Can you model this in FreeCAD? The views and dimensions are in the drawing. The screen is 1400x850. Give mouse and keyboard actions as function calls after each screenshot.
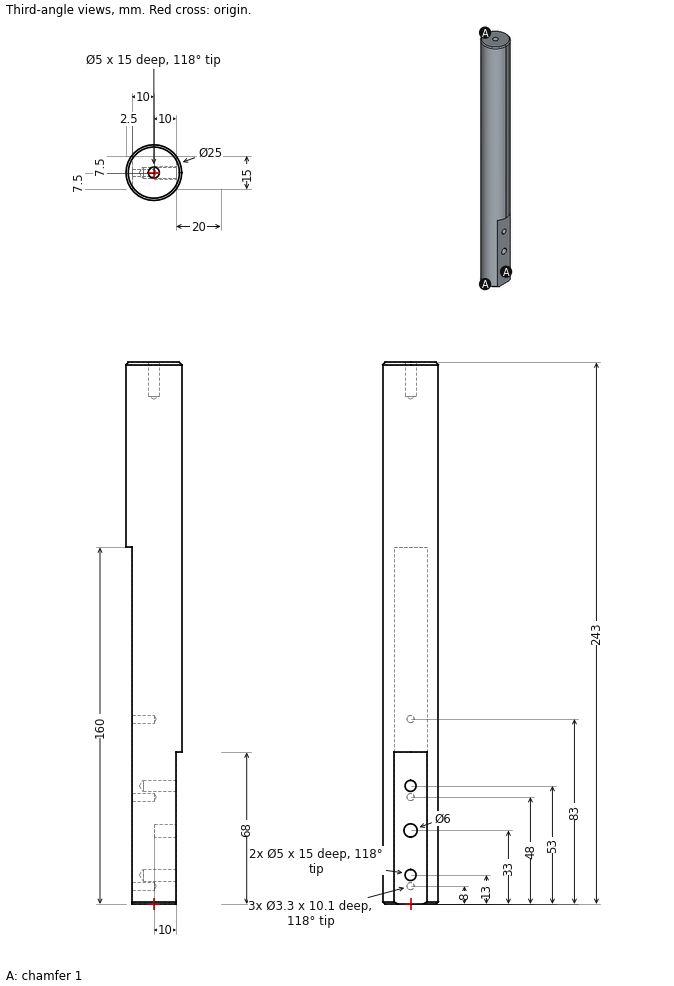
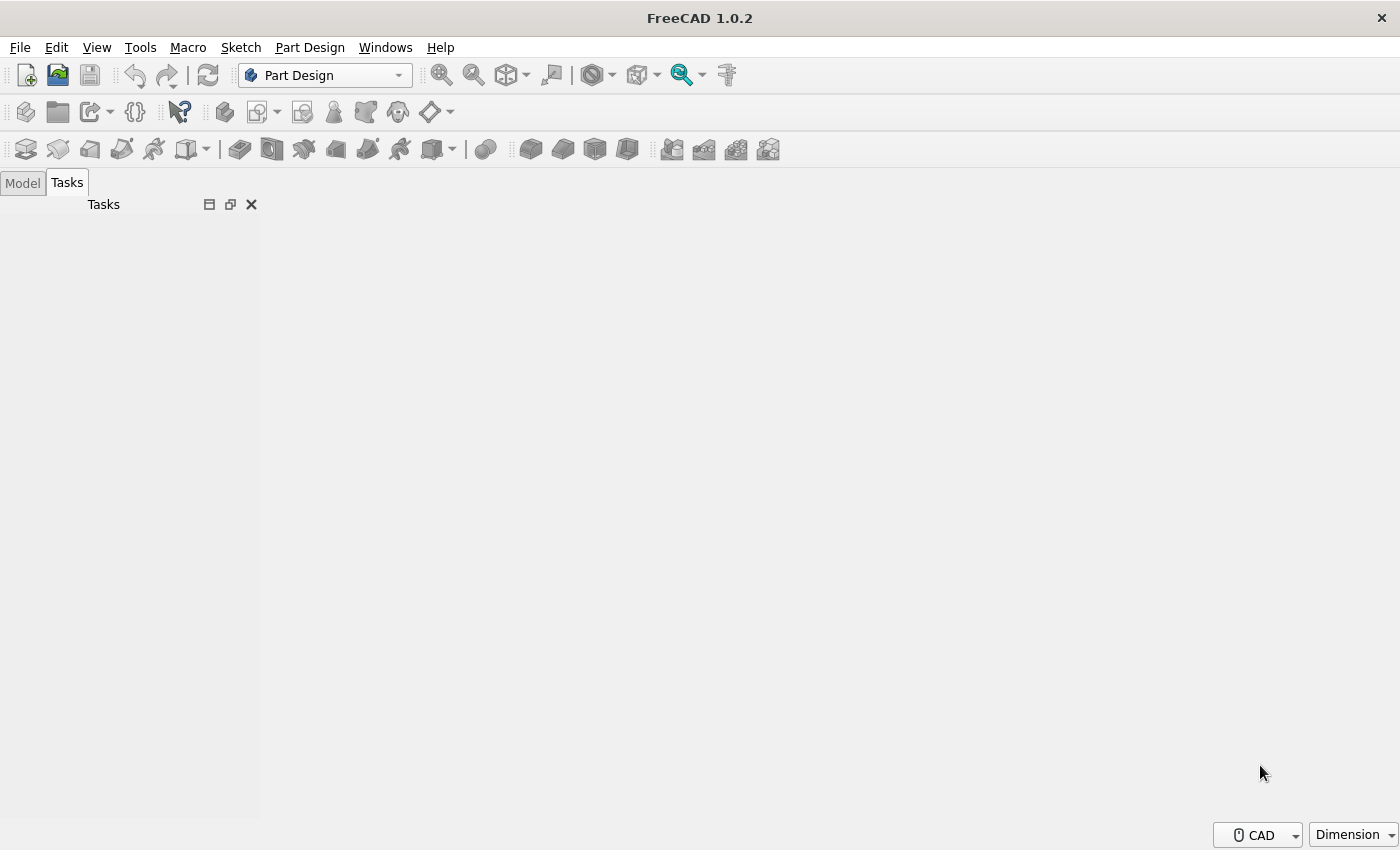
click(26, 76)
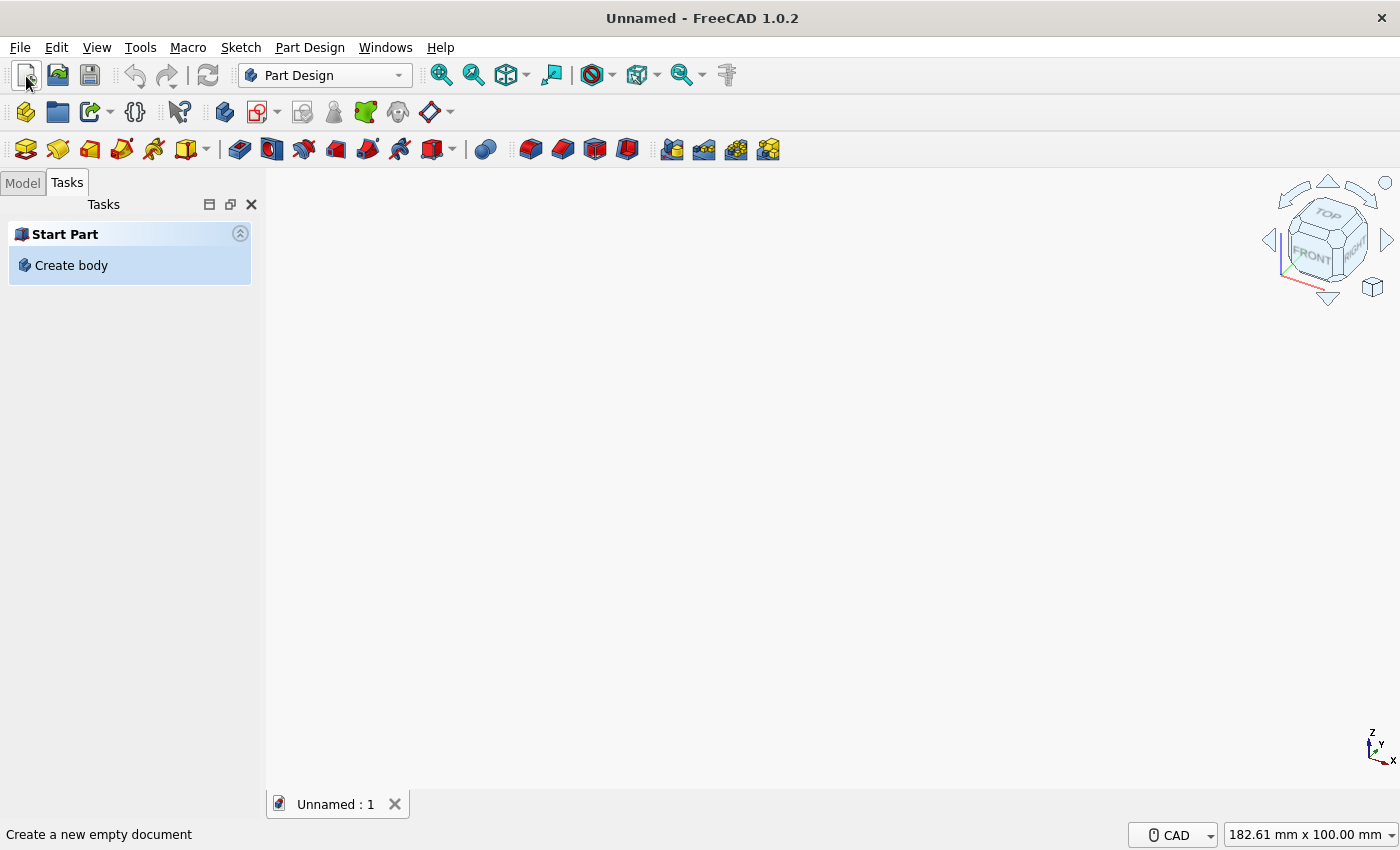
click(258, 112)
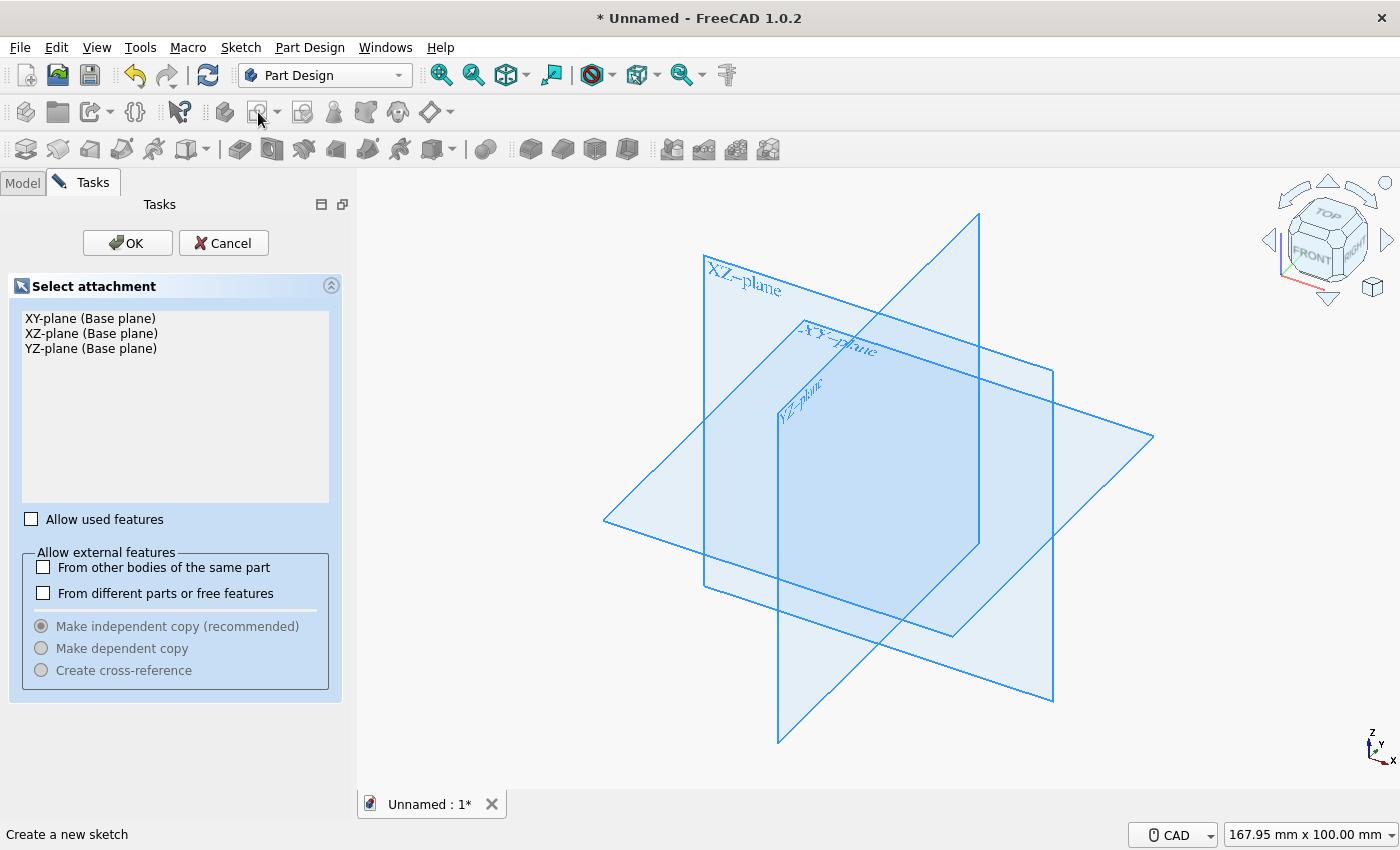
click(82, 318)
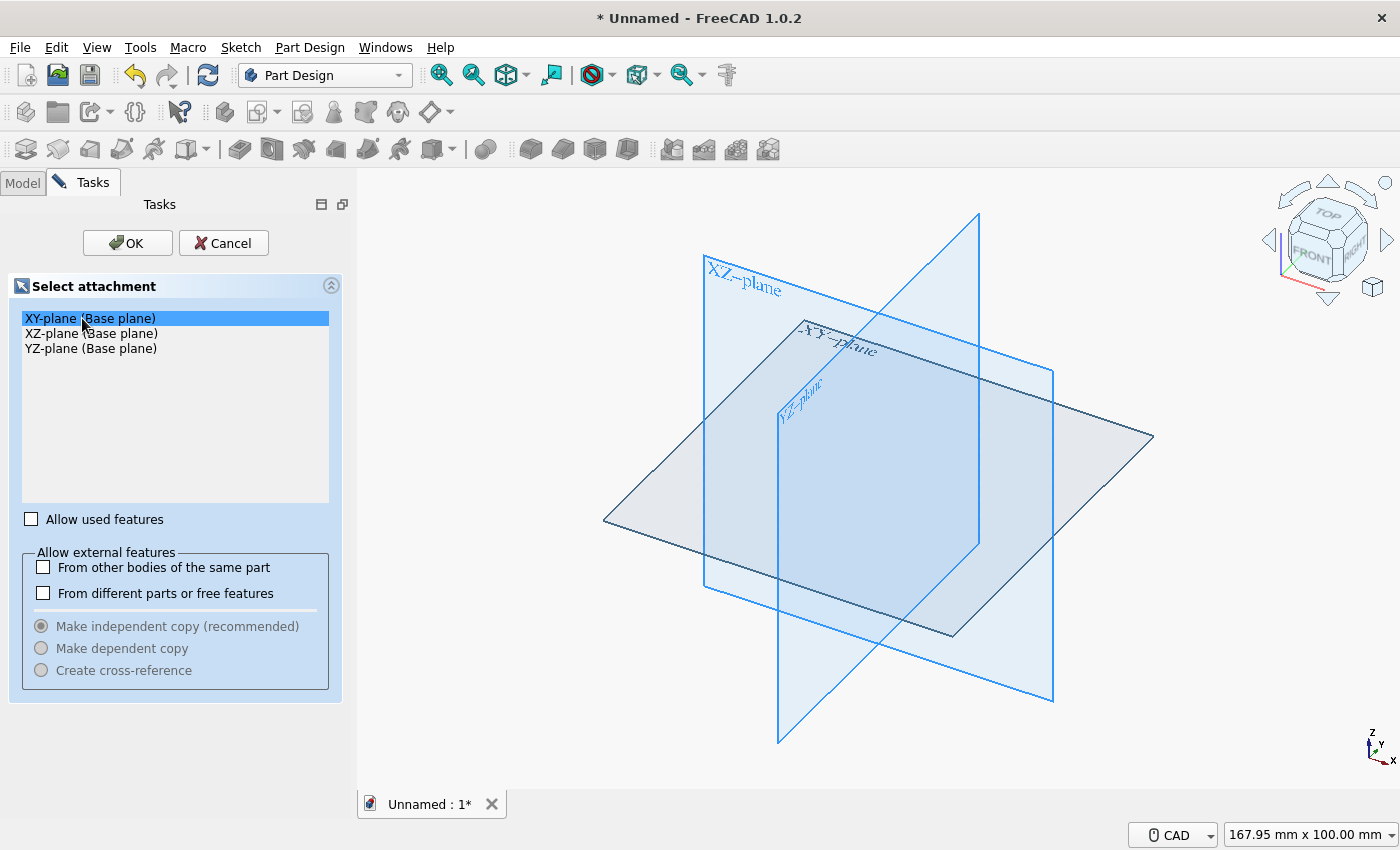
click(128, 243)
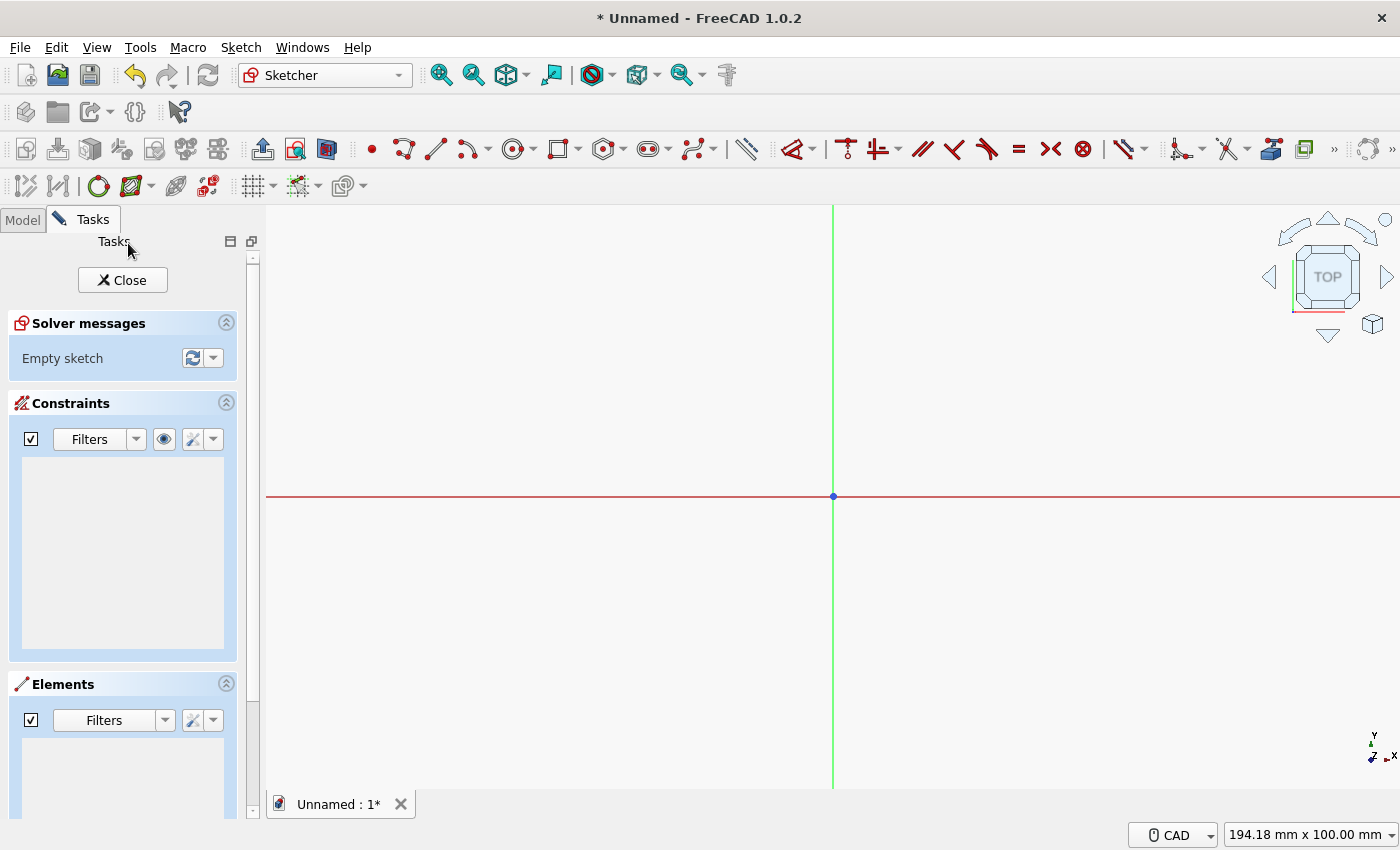
scroll(873, 497, up, 5)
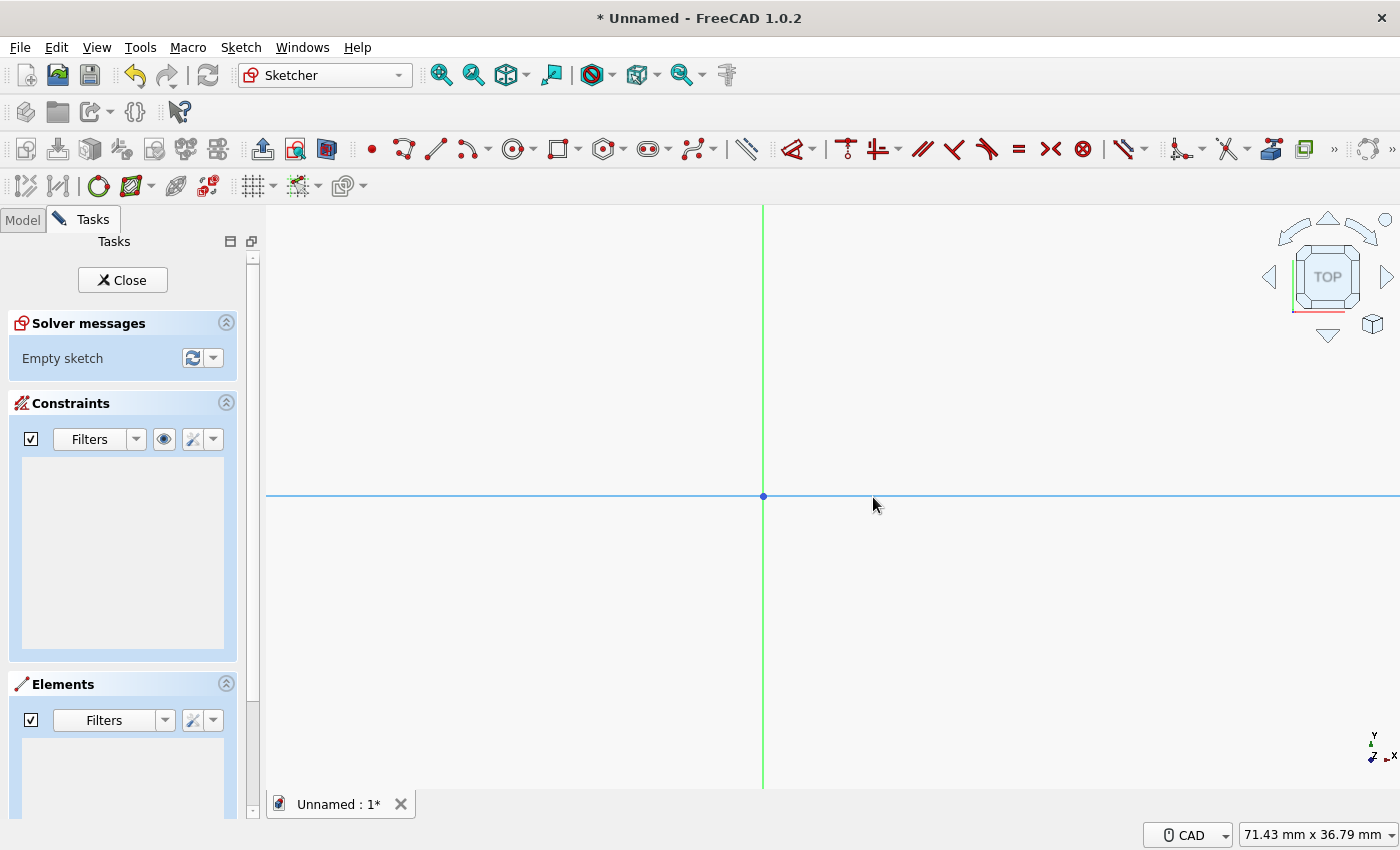
key(g)
key(c)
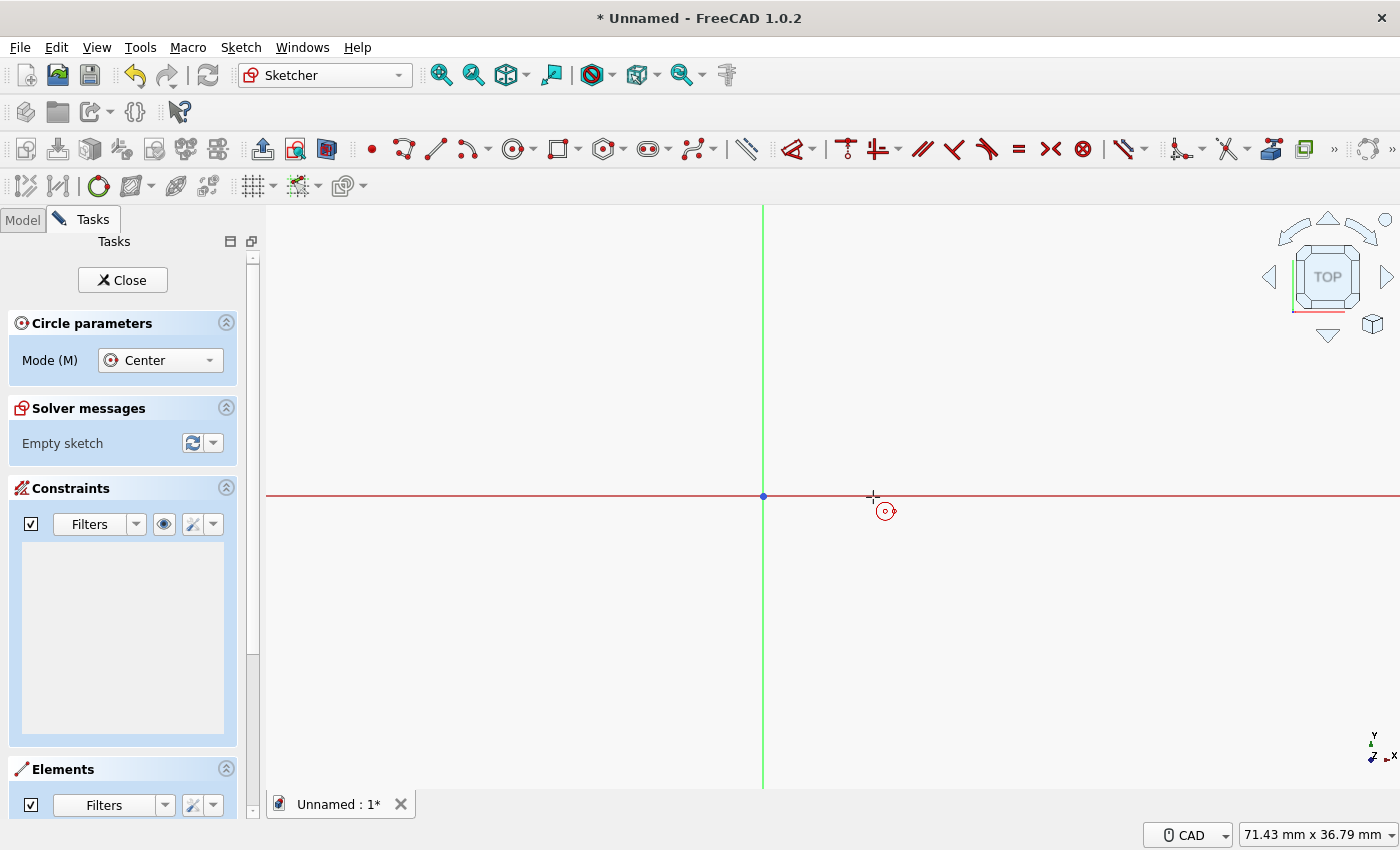
click(763, 496)
click(904, 356)
key(Escape)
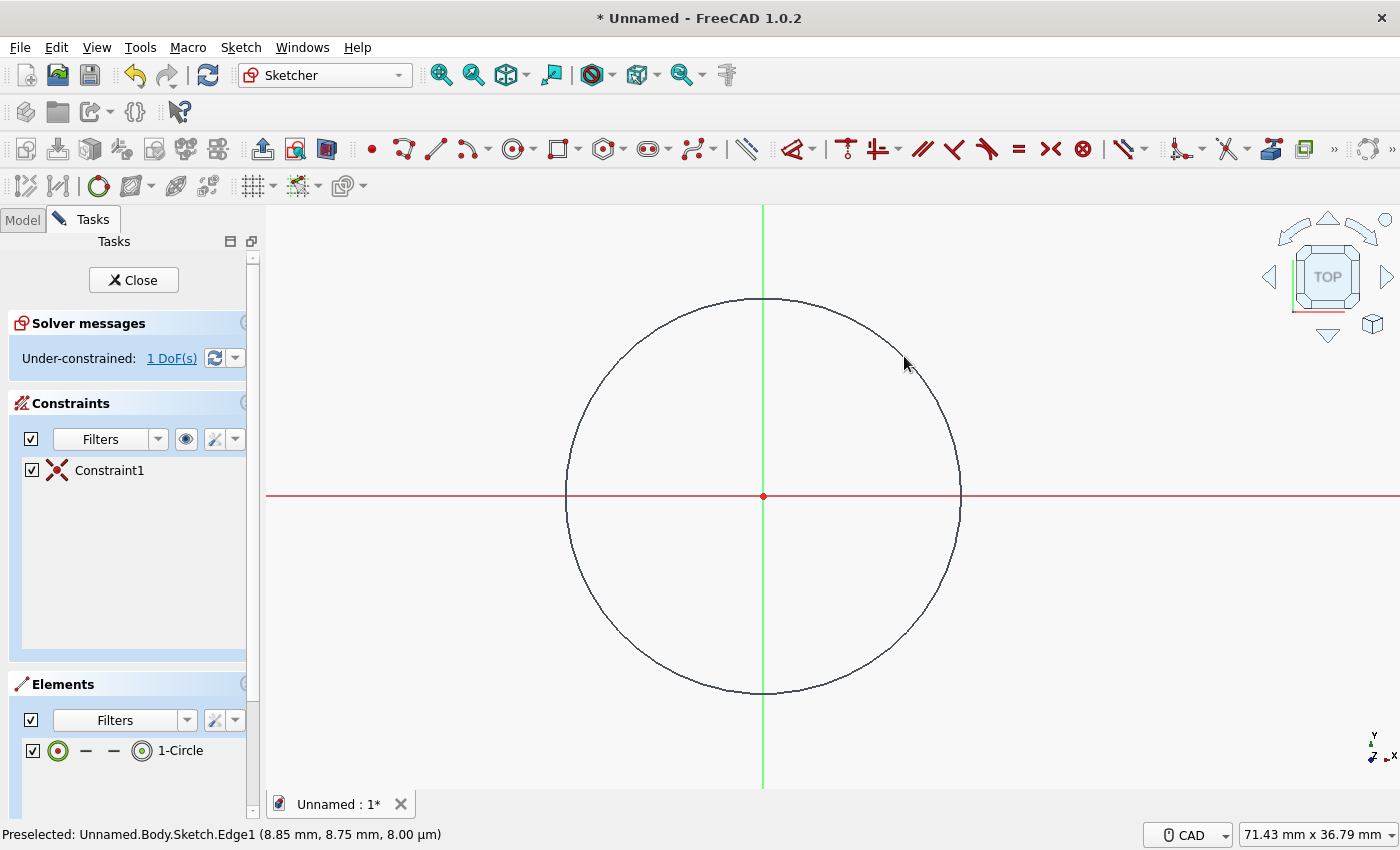
key(d)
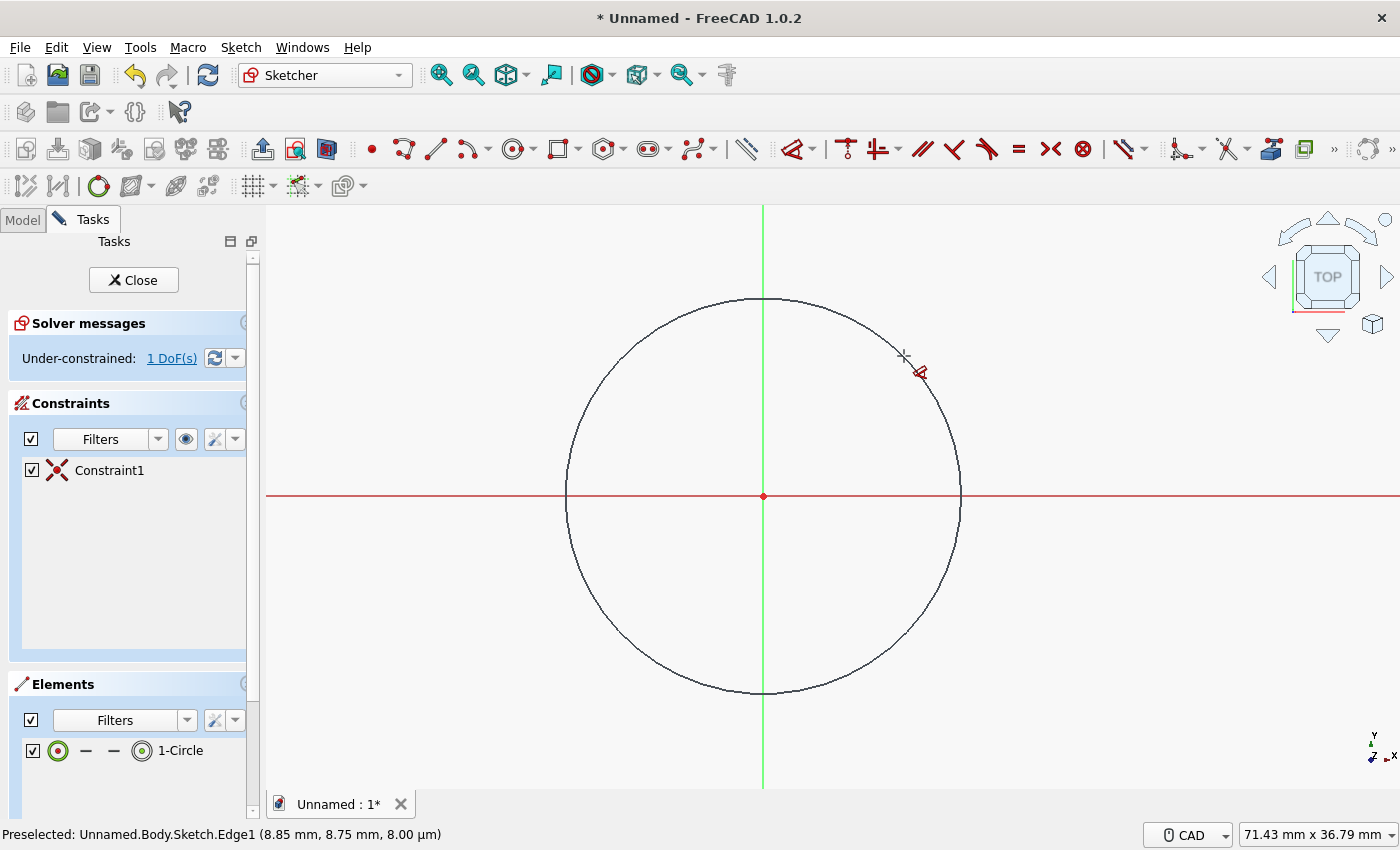
click(903, 356)
click(926, 333)